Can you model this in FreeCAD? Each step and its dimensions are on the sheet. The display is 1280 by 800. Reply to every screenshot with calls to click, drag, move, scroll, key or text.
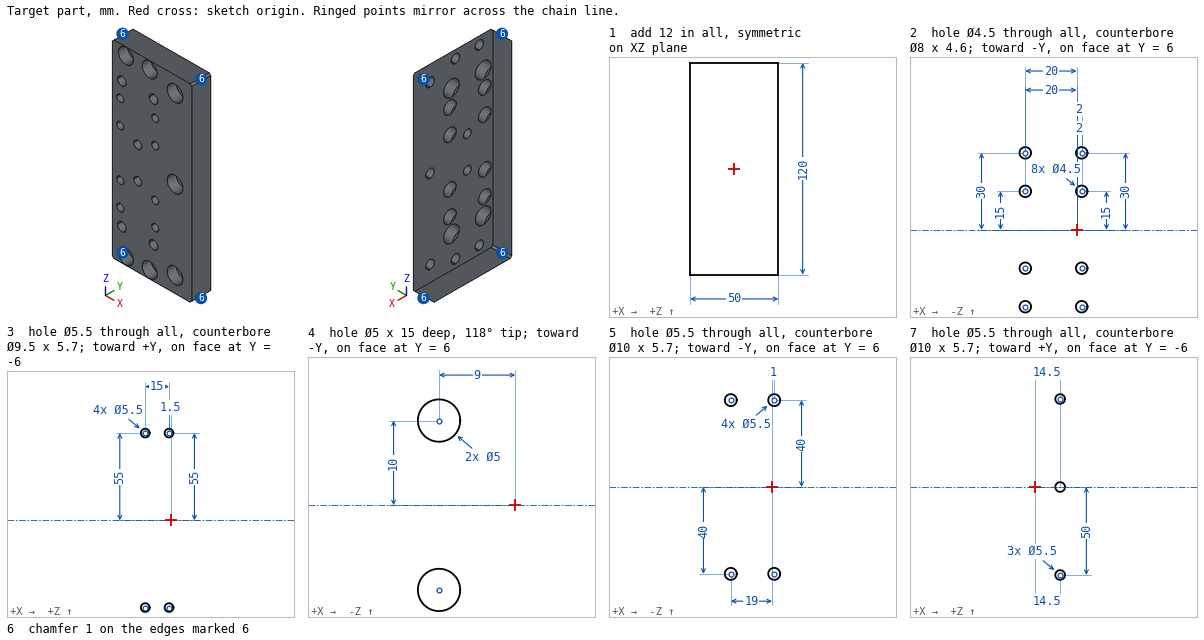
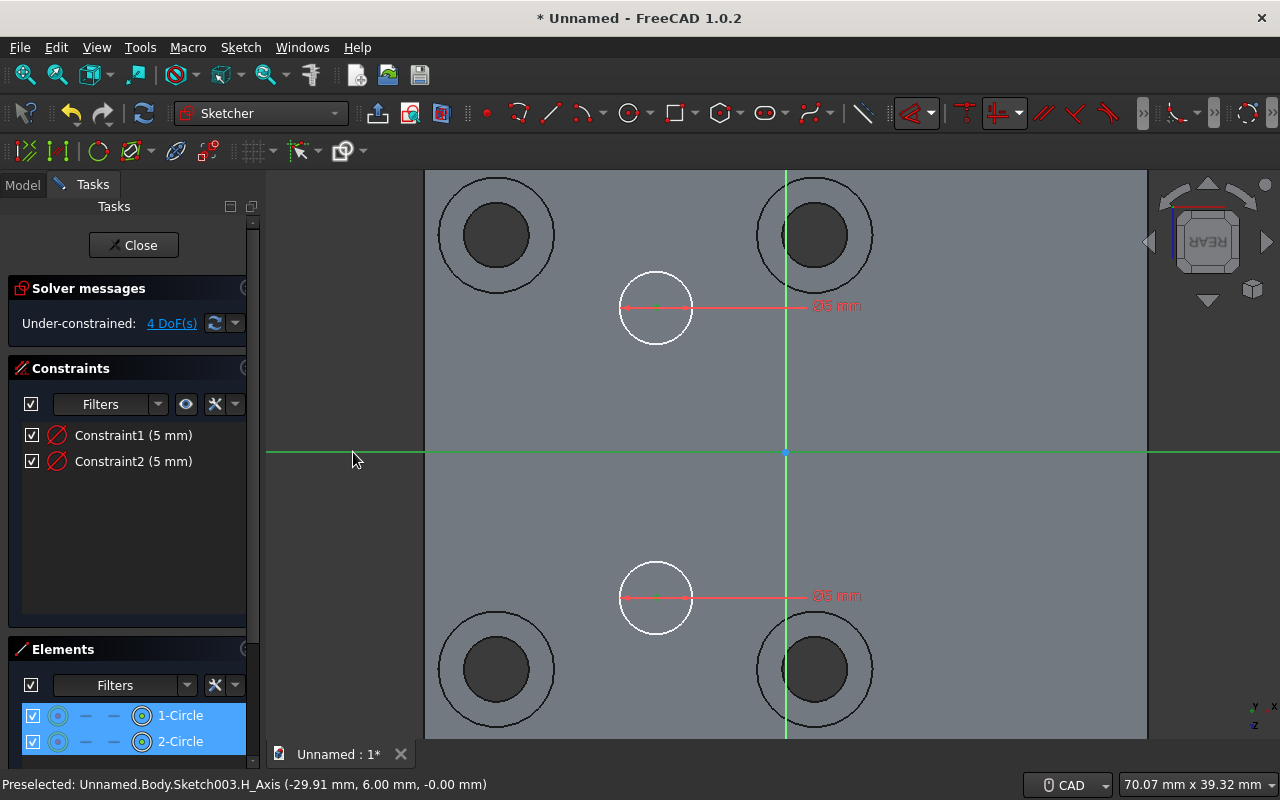
key(s)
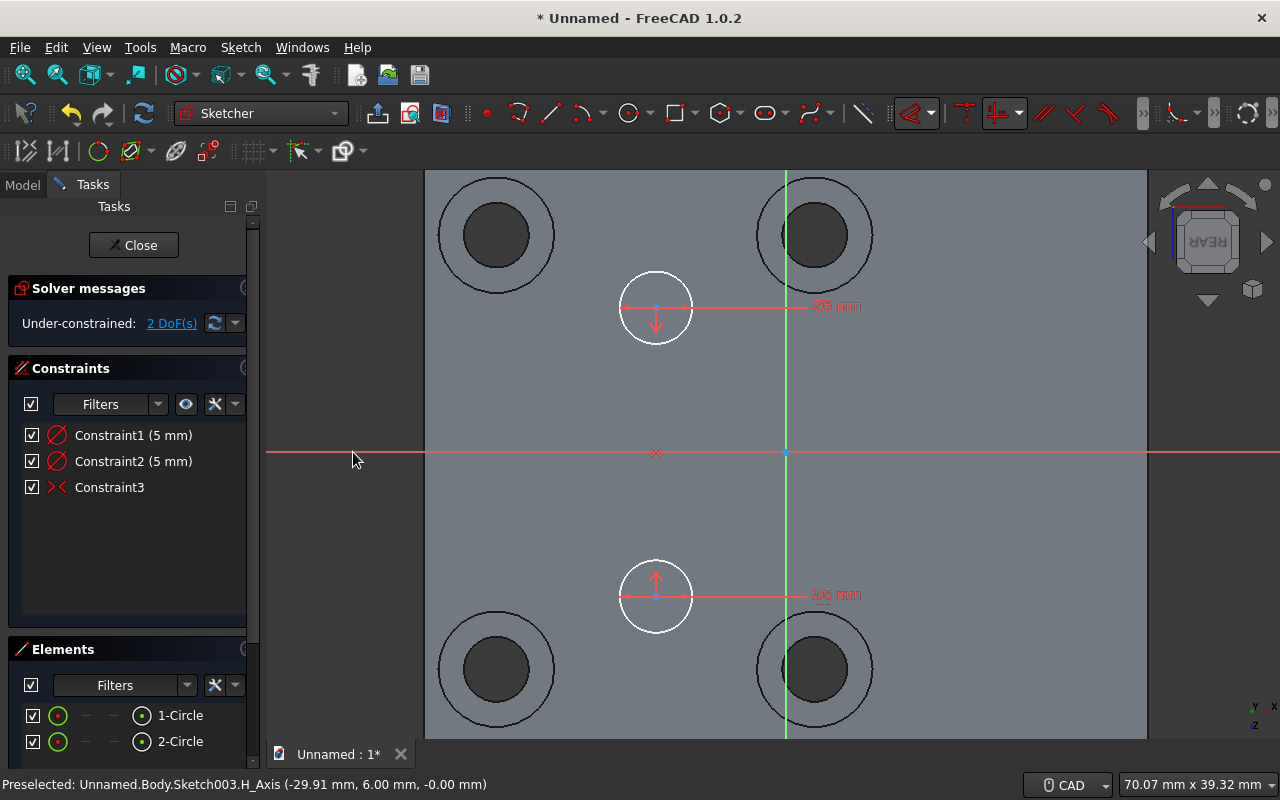
click(656, 308)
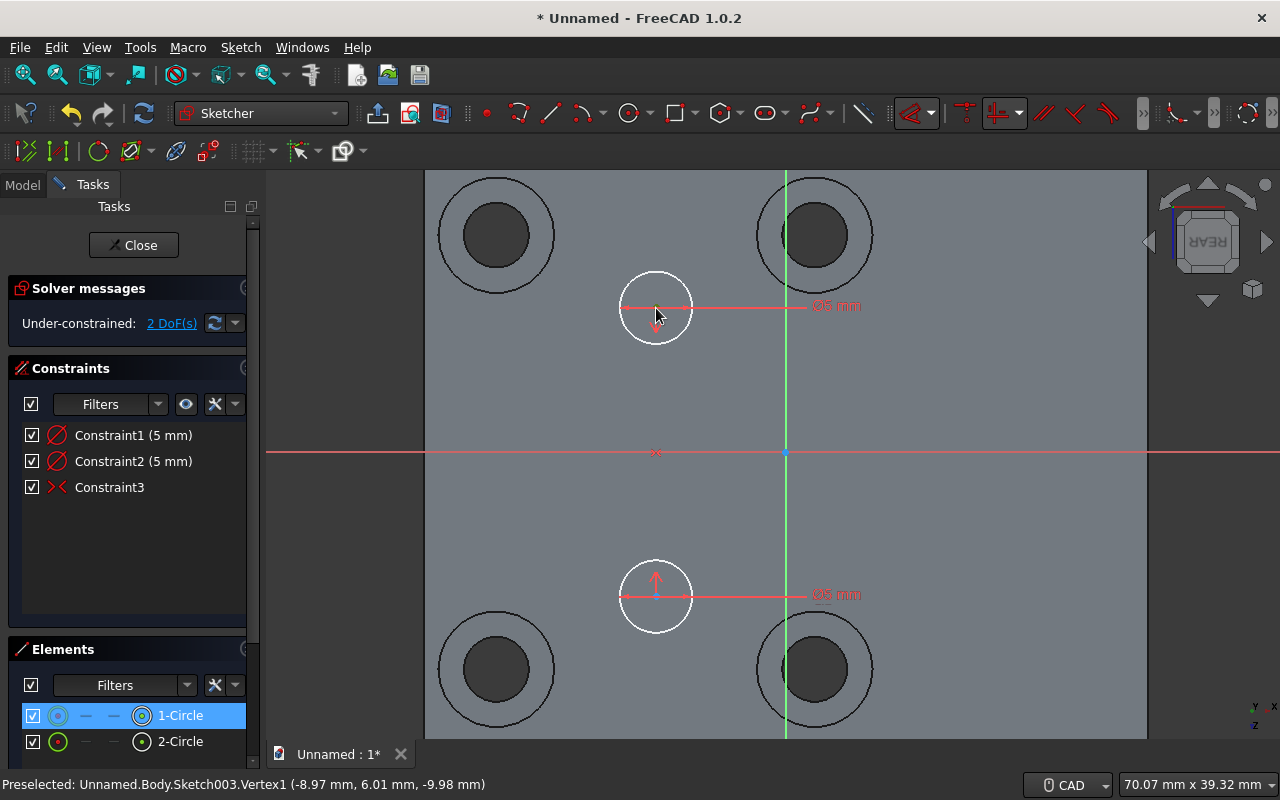
click(934, 114)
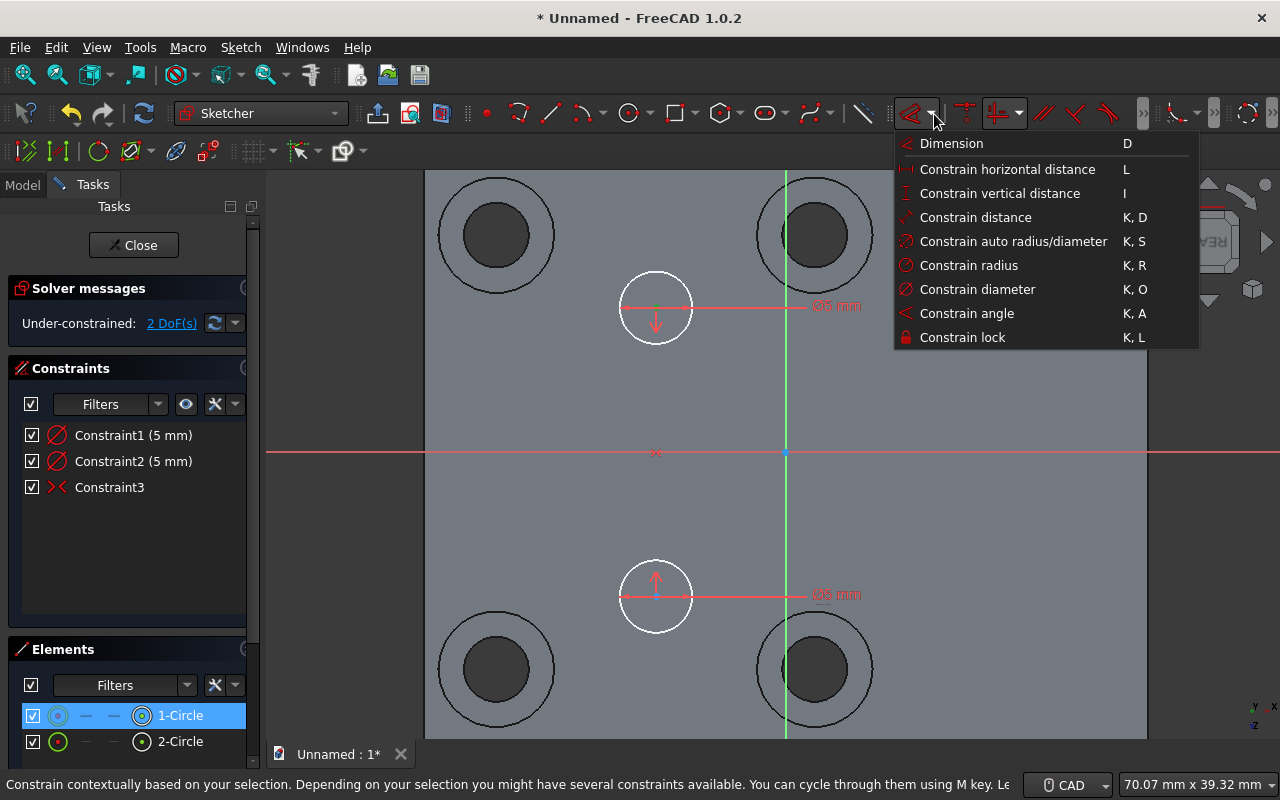
click(1047, 169)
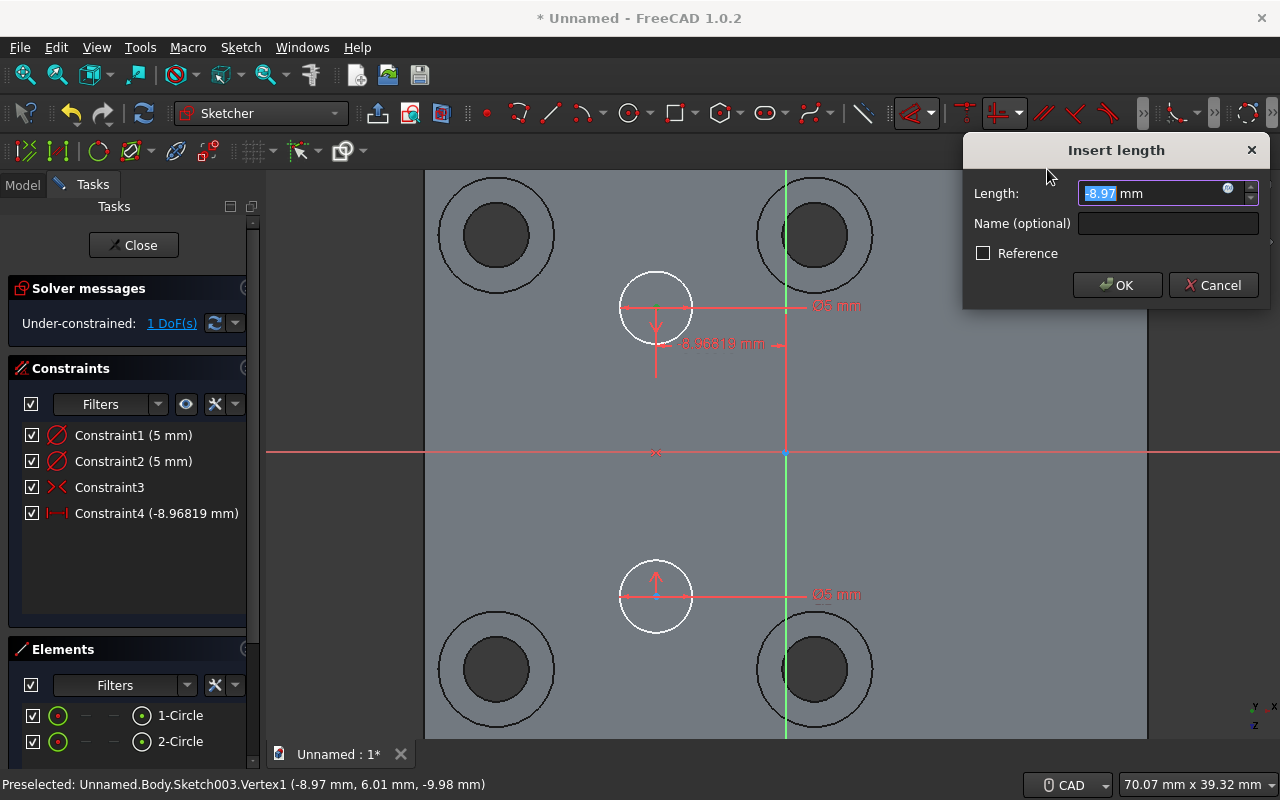
text(-9)
key(Return)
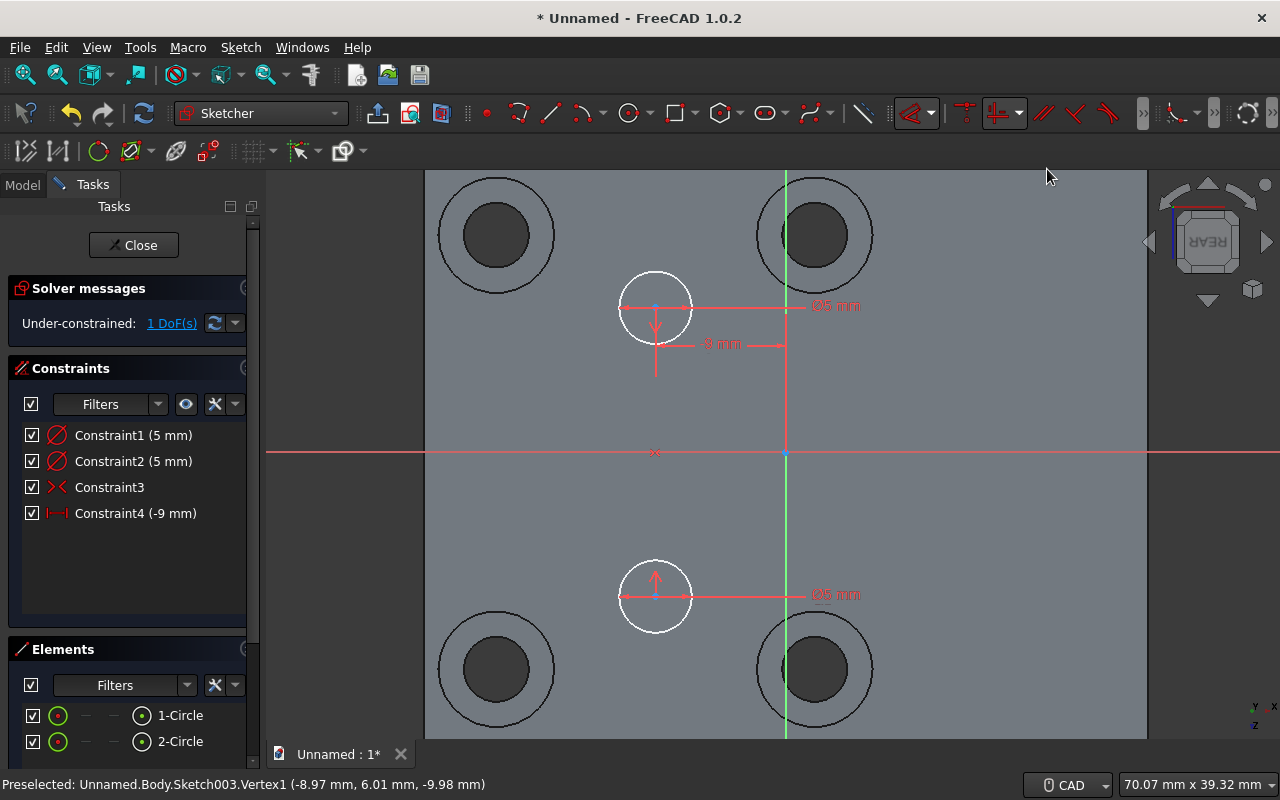
click(656, 308)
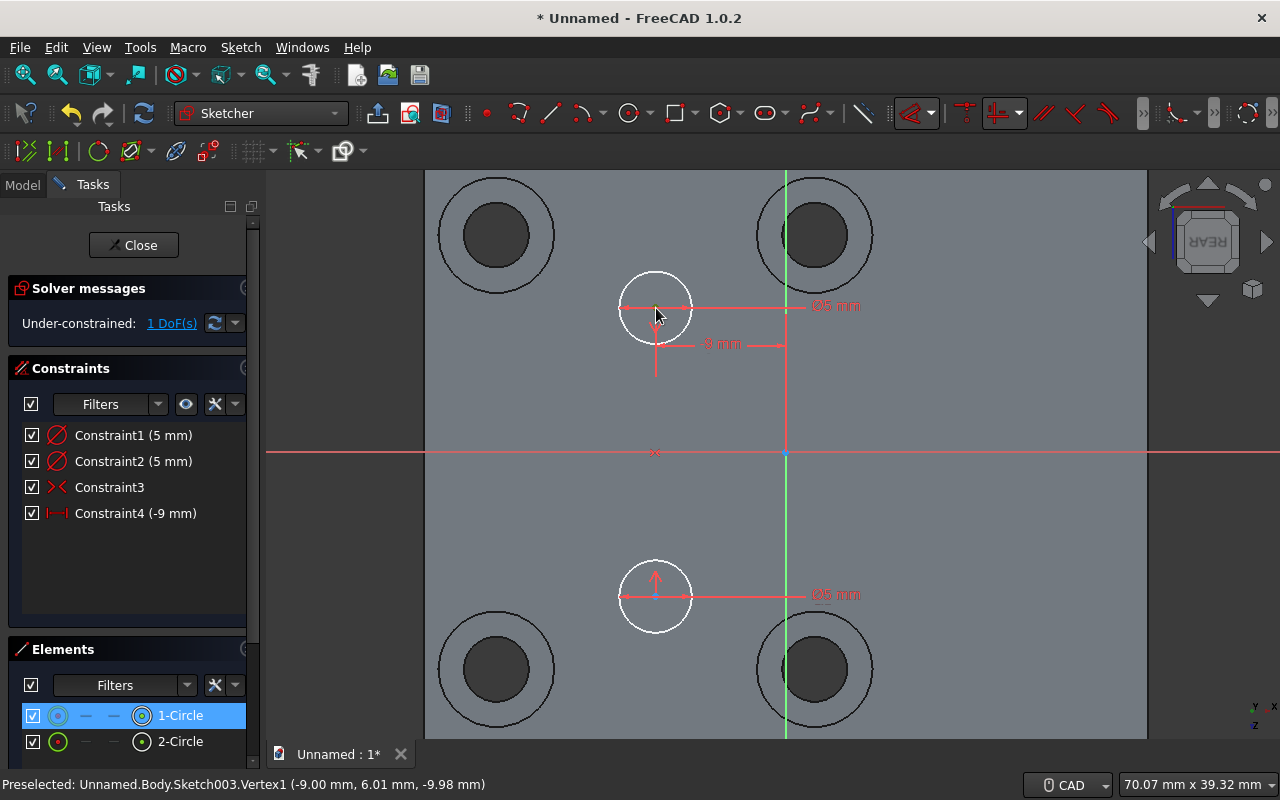
click(934, 114)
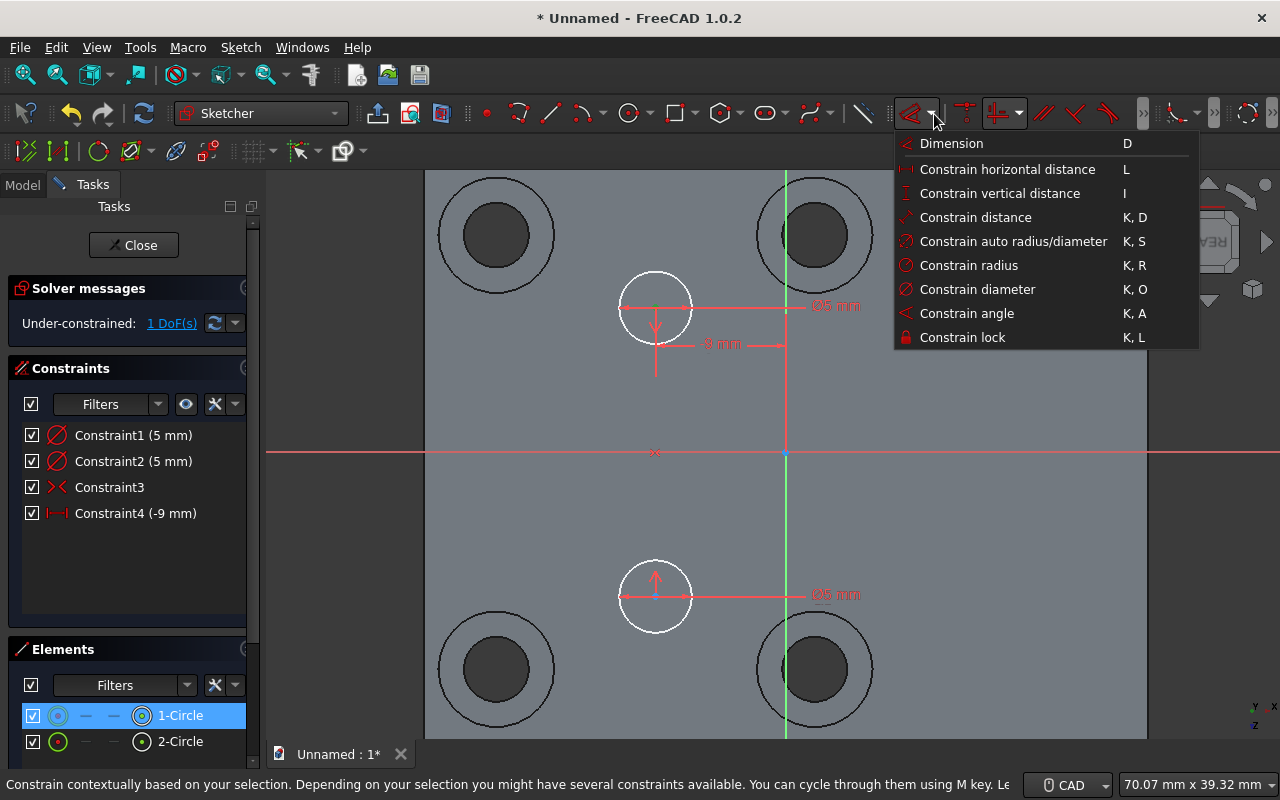
click(1047, 193)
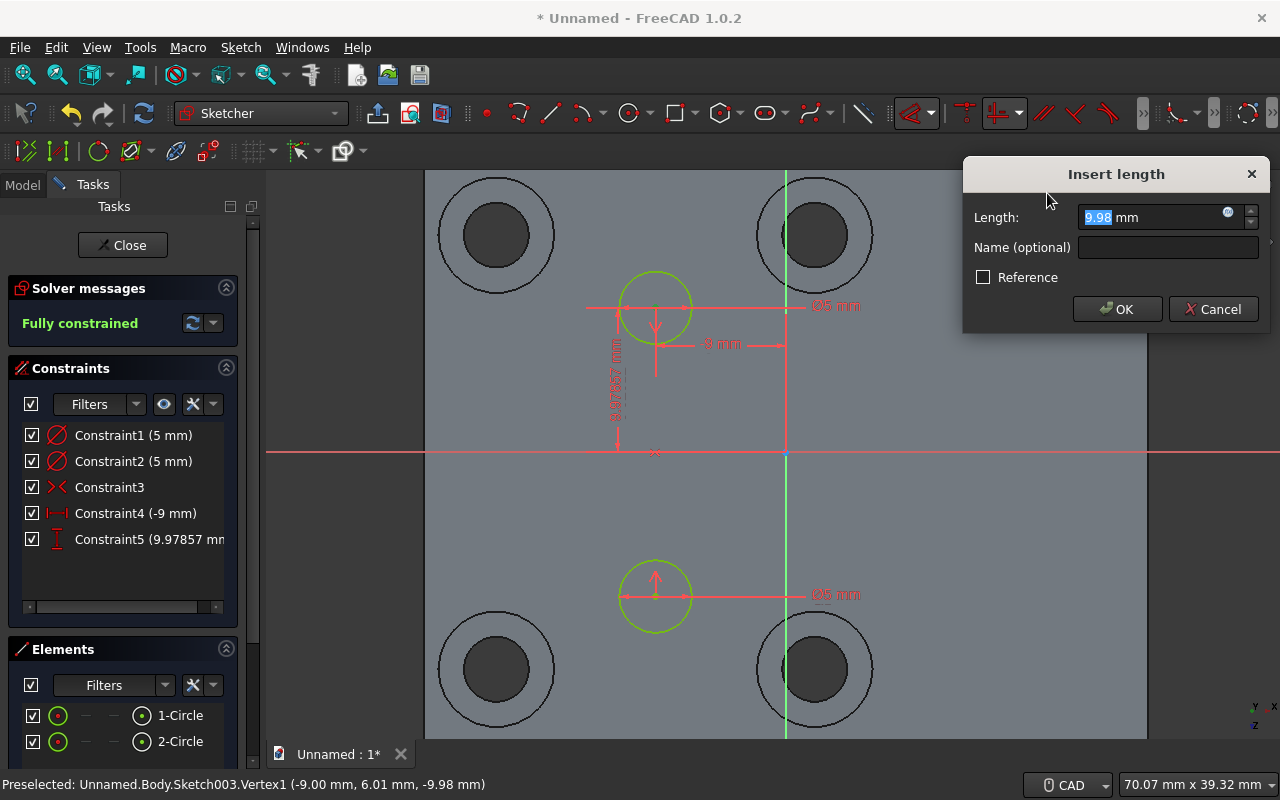
text(10)
key(Return)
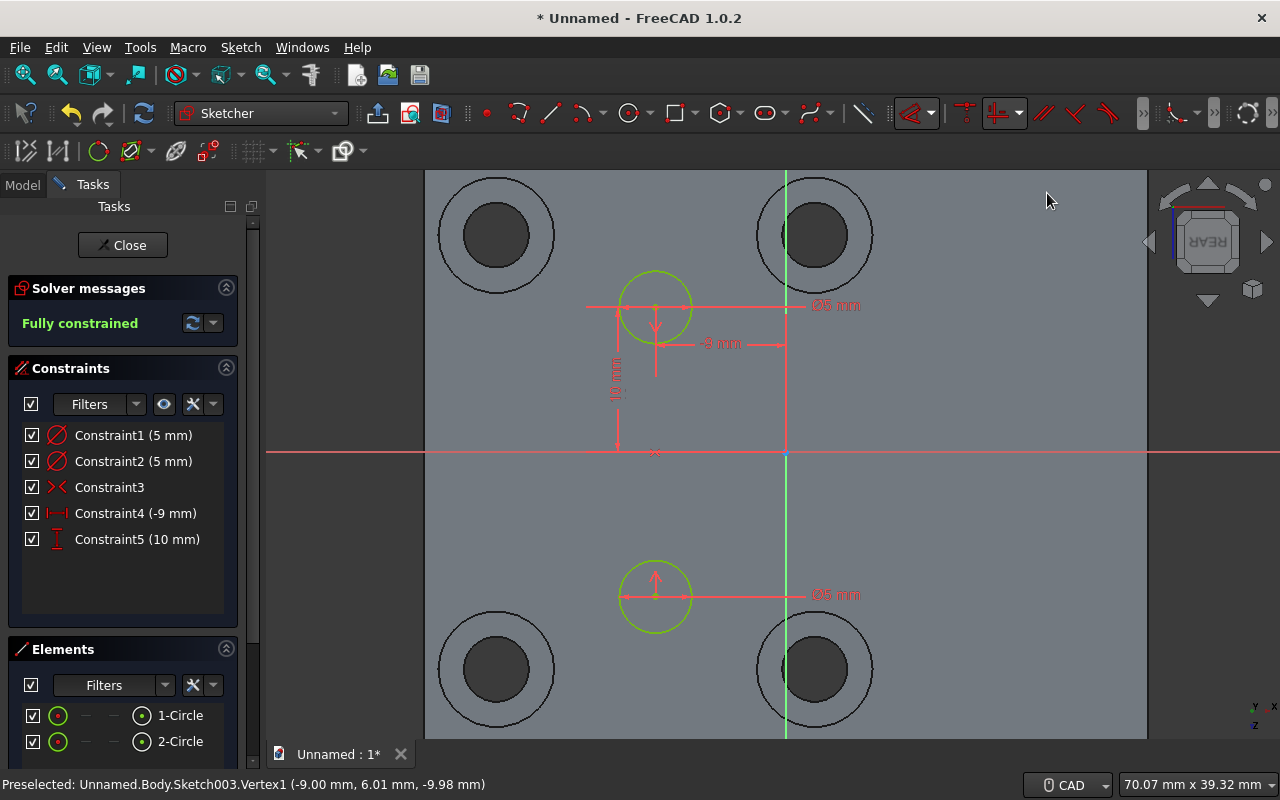
click(123, 245)